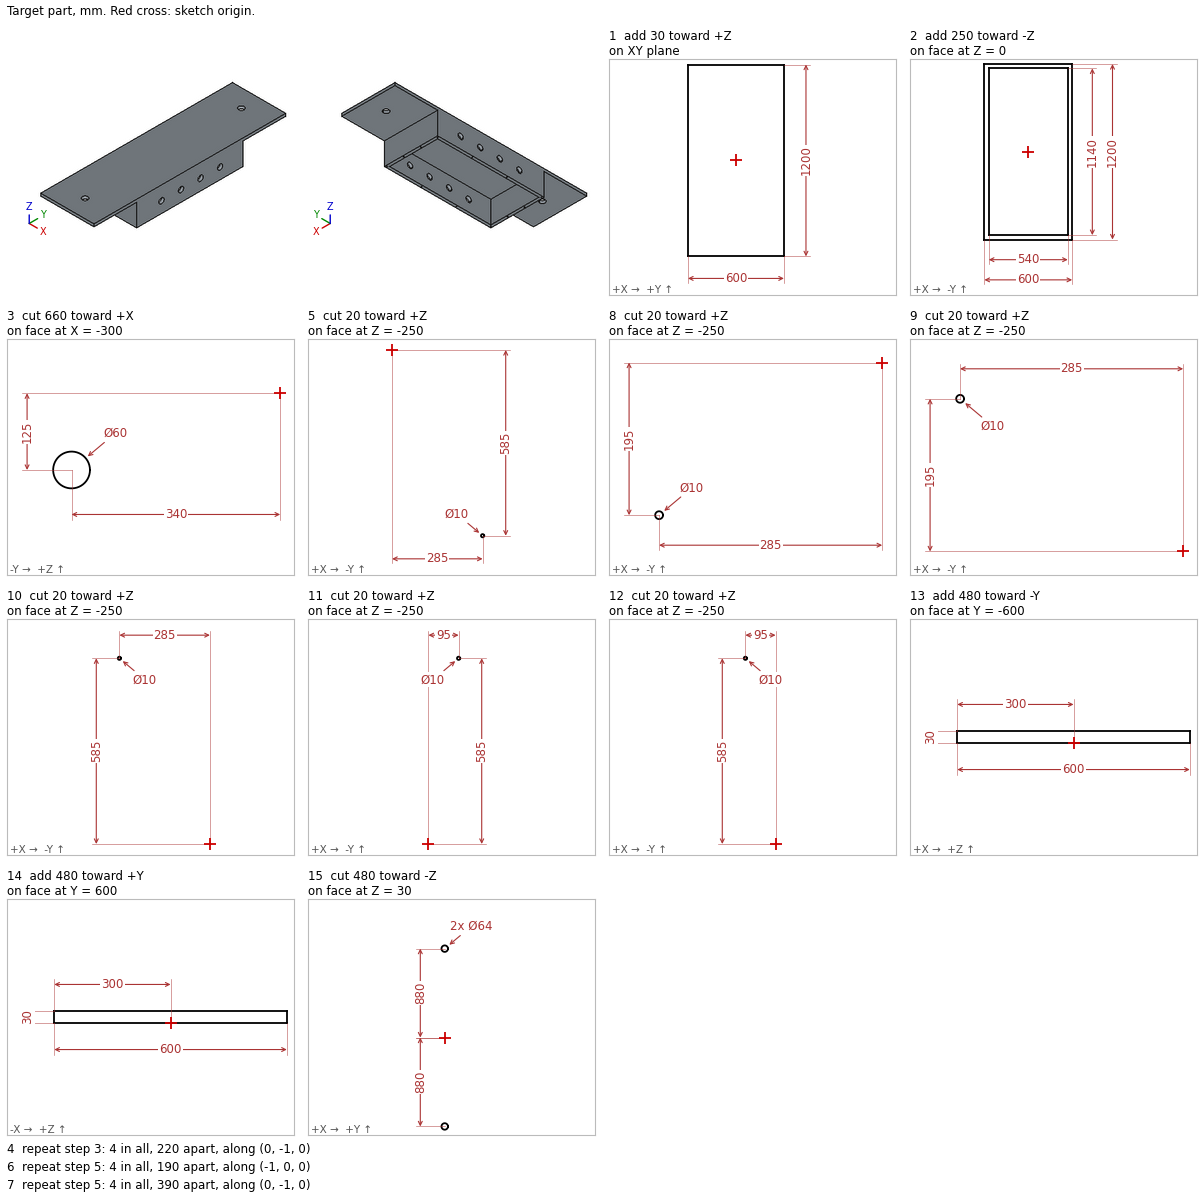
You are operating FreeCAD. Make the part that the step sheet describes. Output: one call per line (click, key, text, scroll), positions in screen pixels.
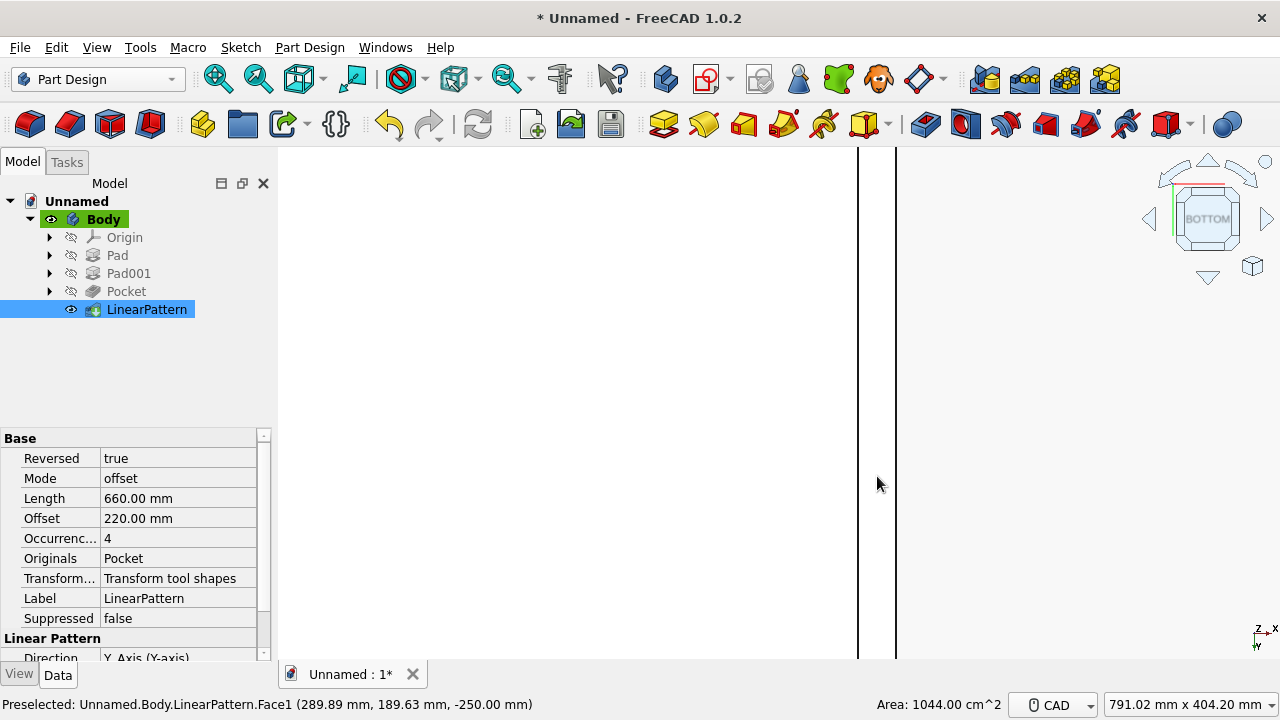
click(706, 80)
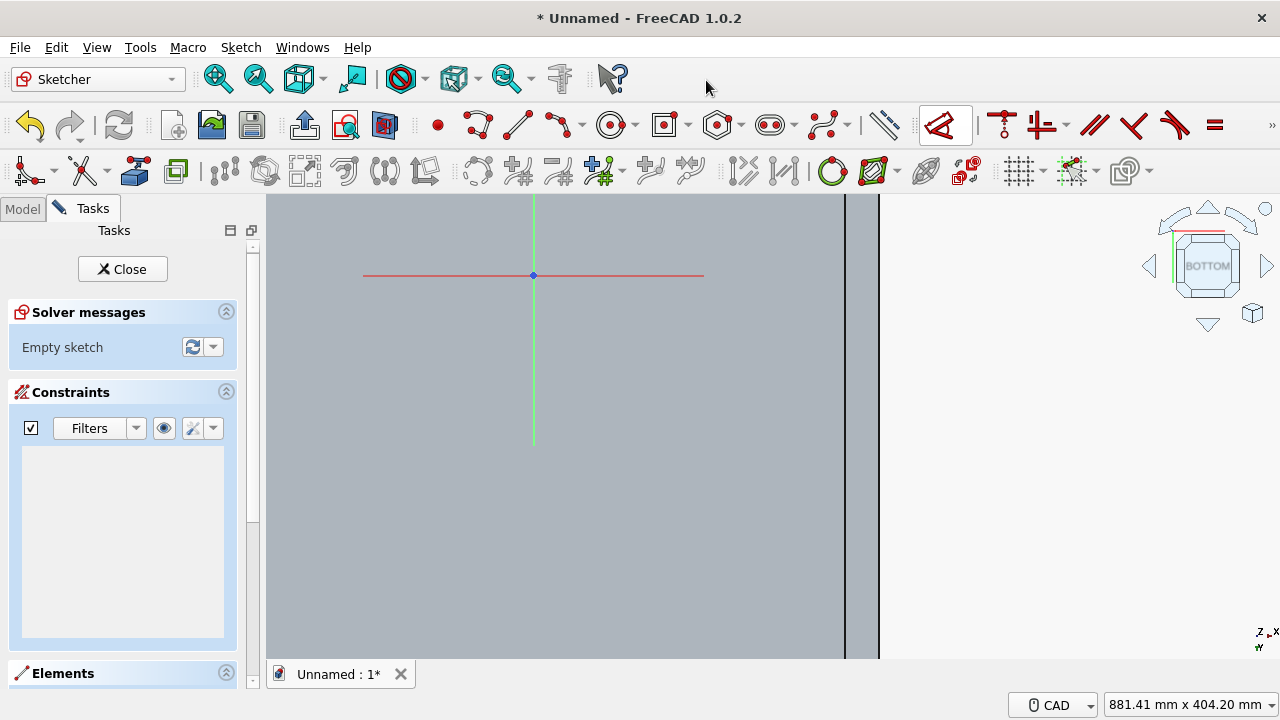
scroll(704, 426, down, 5)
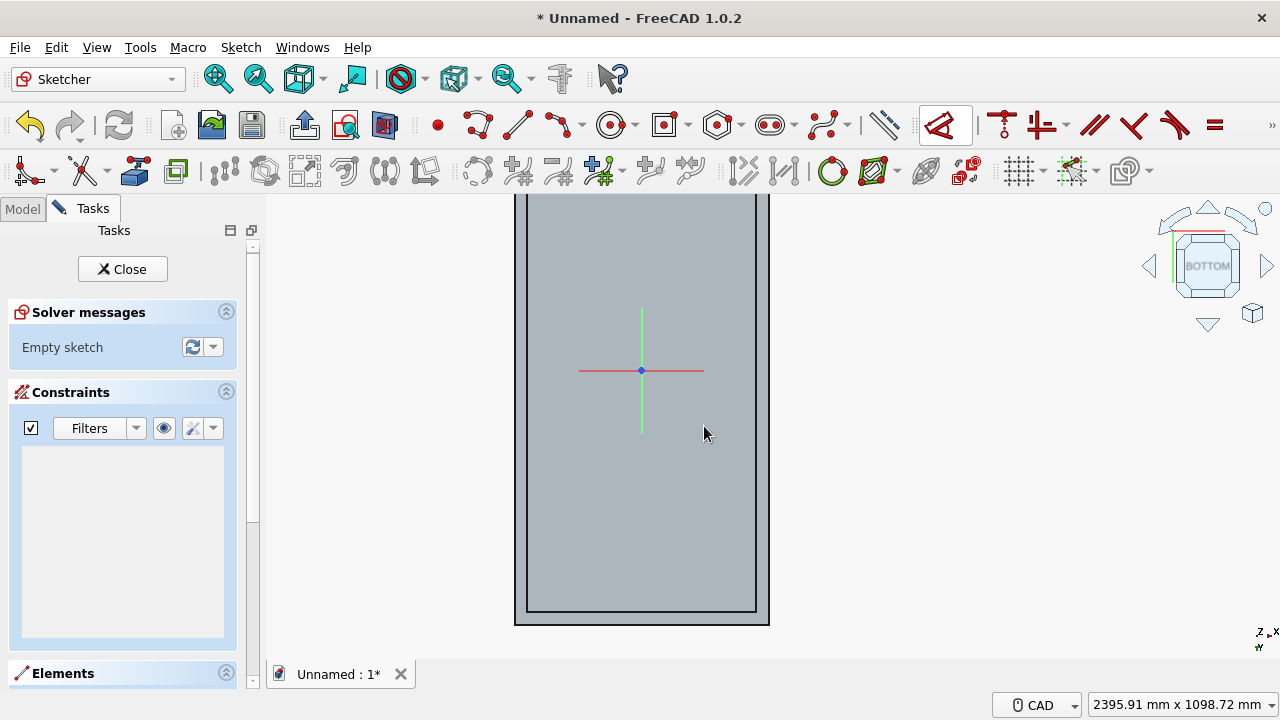
scroll(765, 629, up, 15)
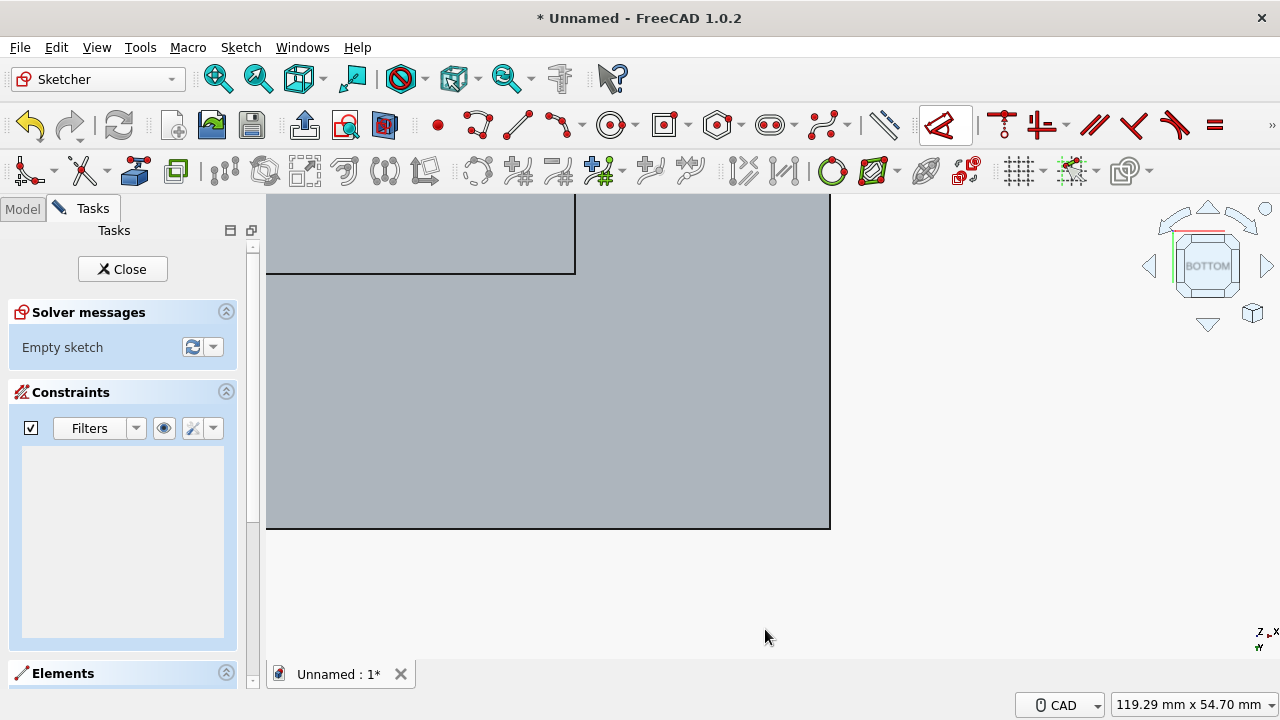
scroll(701, 390, up, 6)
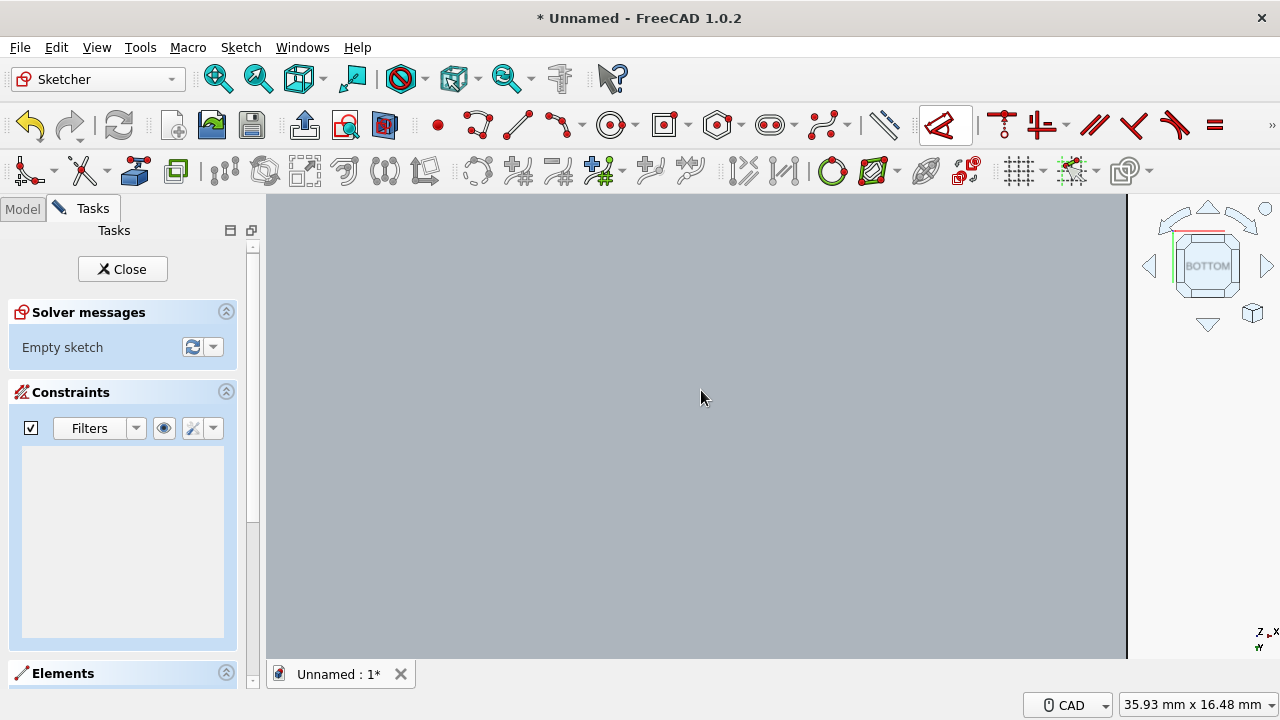
click(612, 126)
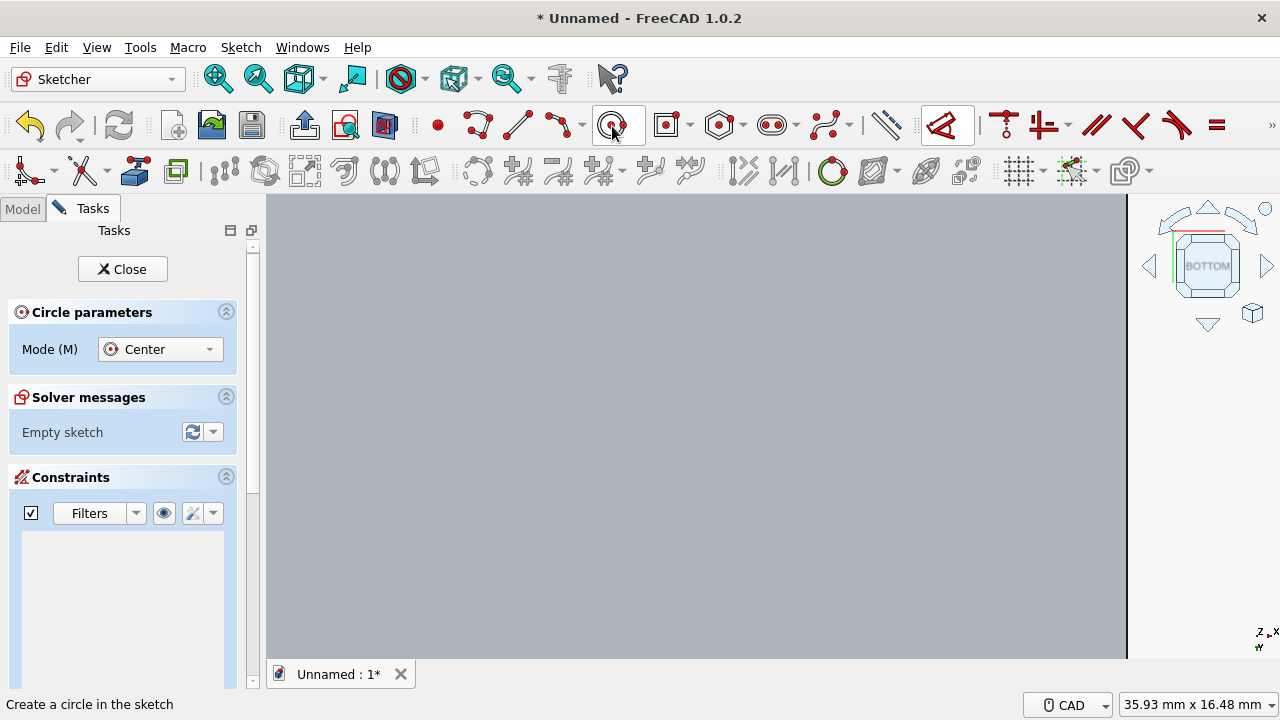
click(703, 426)
move(803, 327)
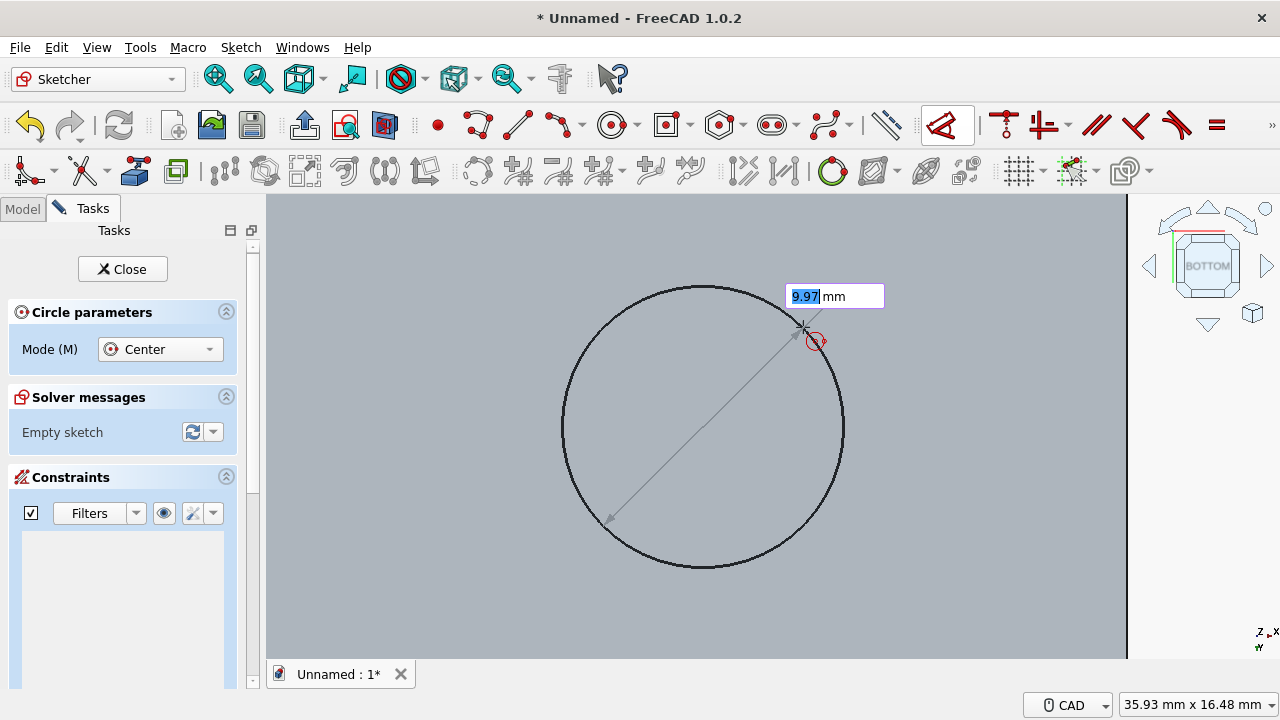
text(10)
key(Return)
key(Escape)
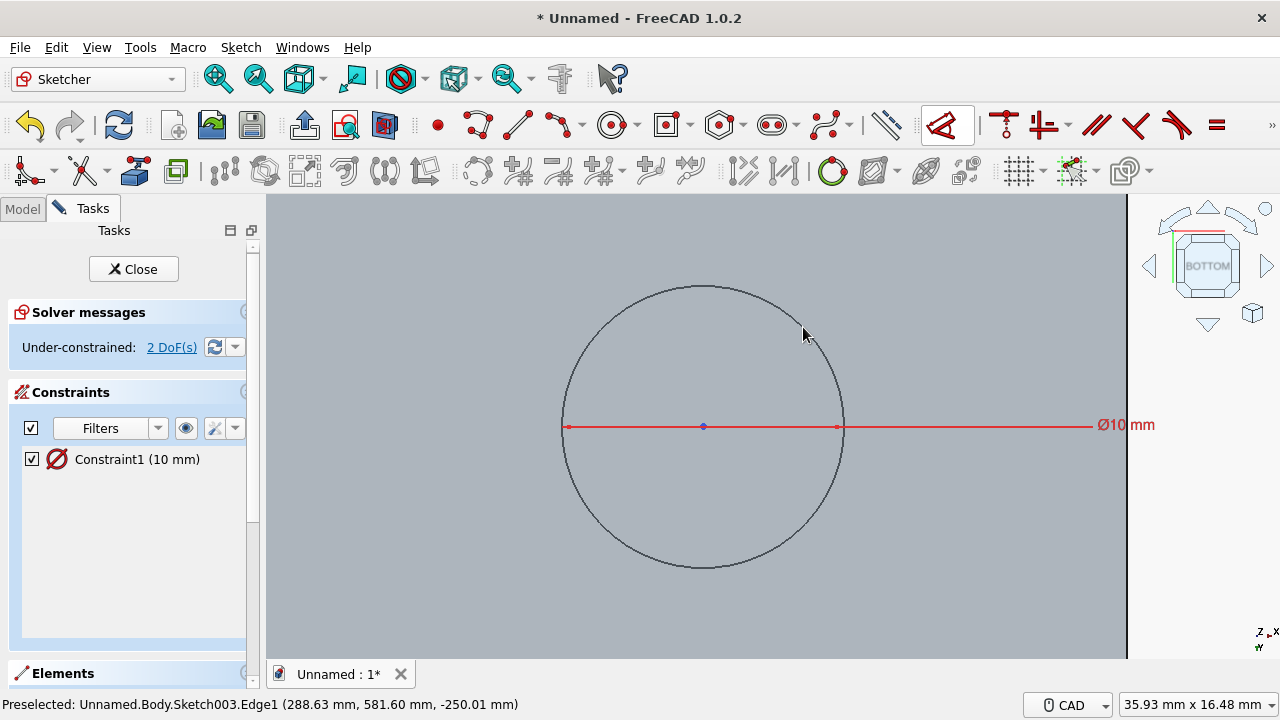
click(703, 427)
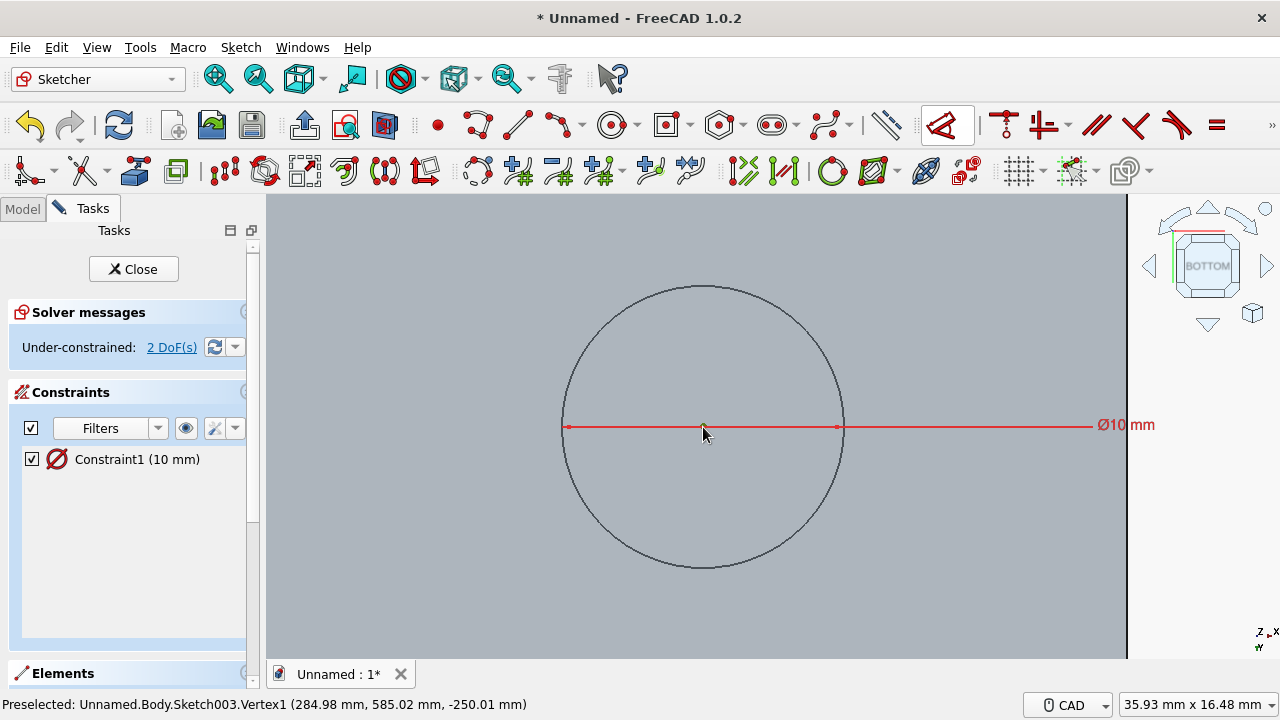
click(968, 126)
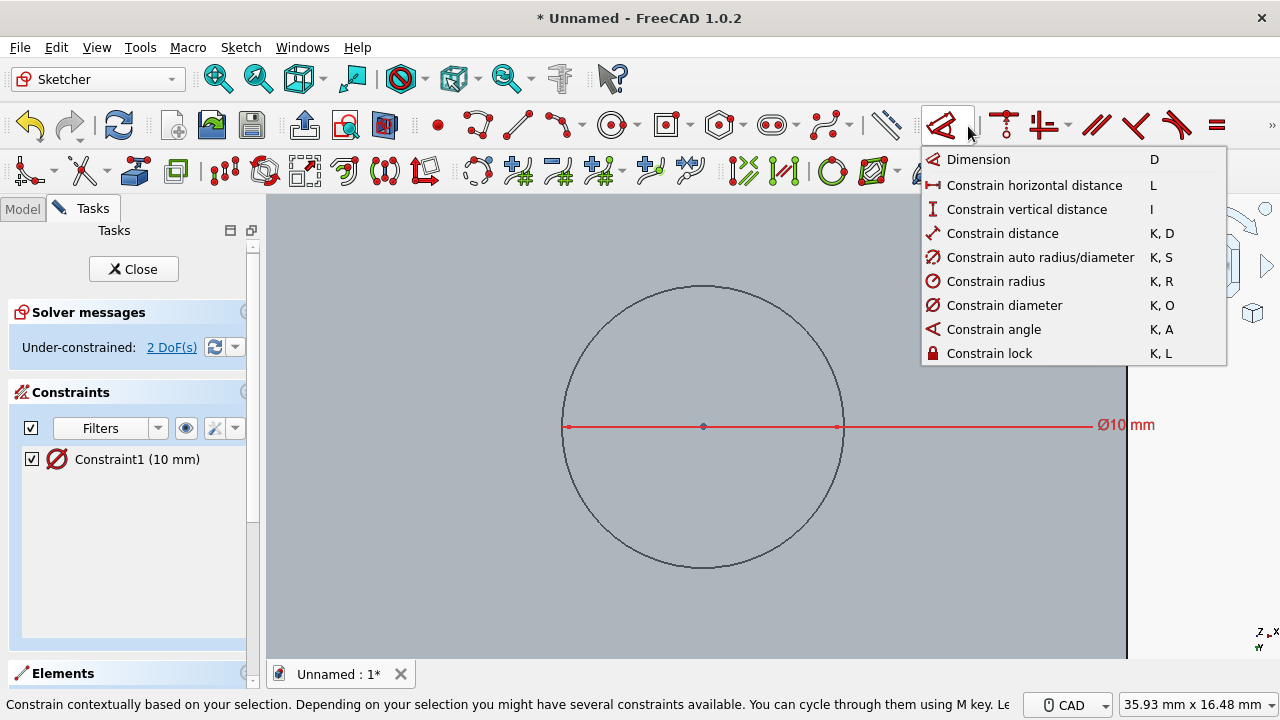
click(1074, 185)